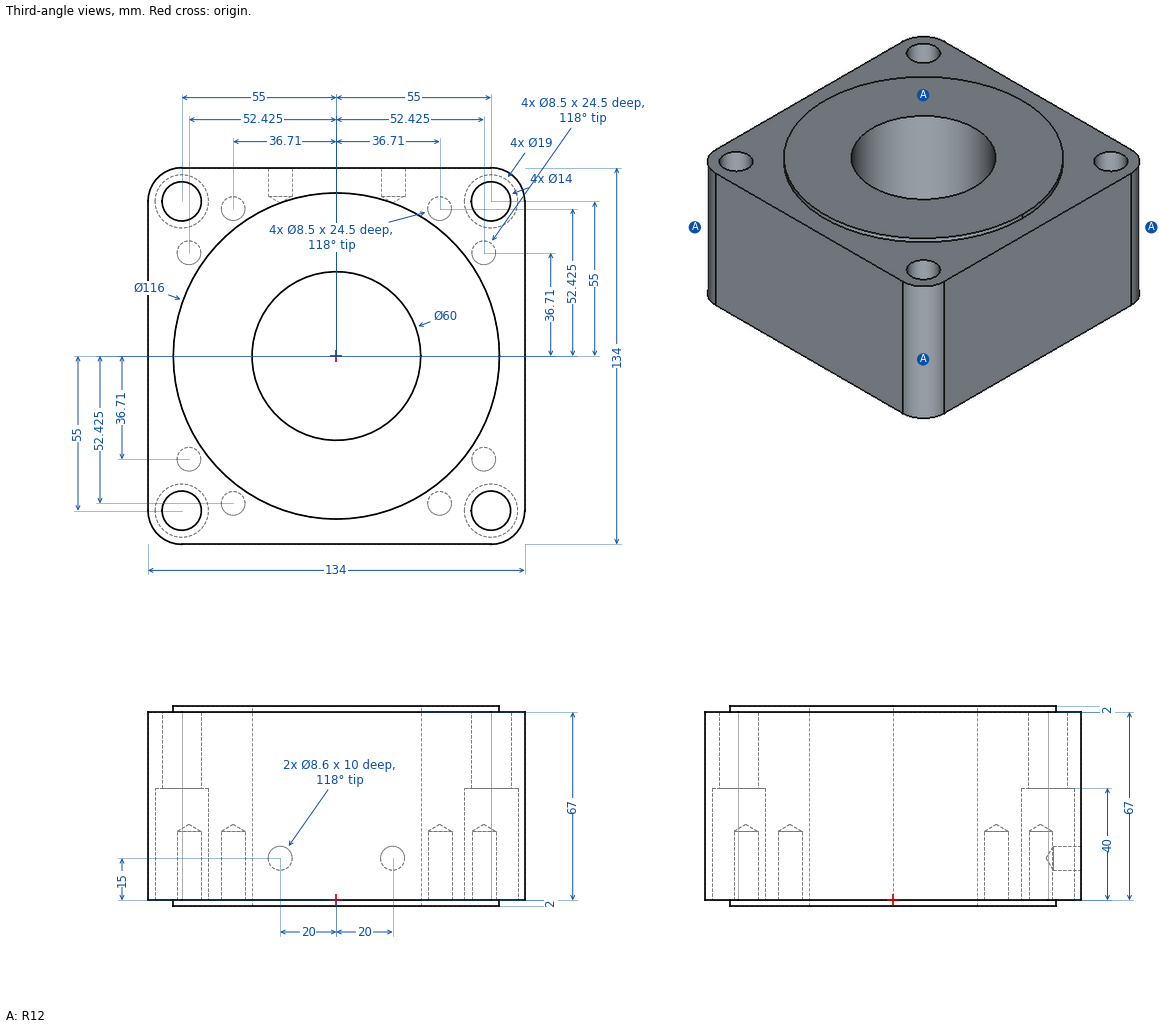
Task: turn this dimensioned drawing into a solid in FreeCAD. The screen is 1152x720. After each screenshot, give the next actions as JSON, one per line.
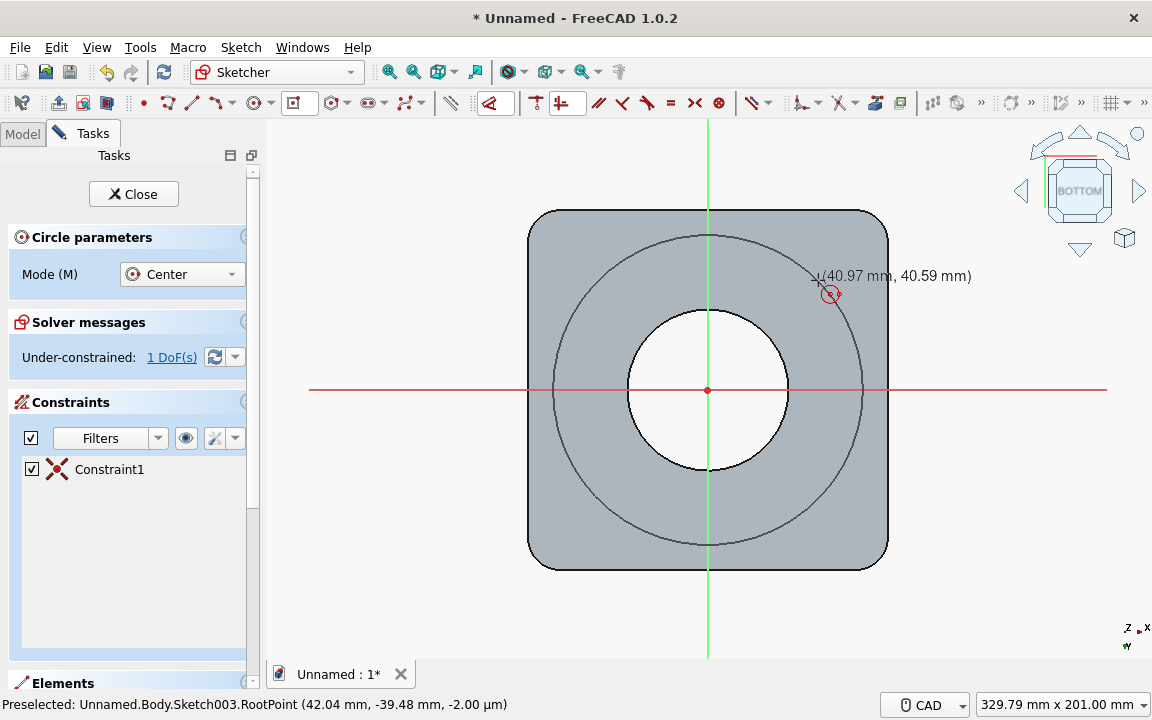
{"action": "left_click", "coordinate": [708, 390]}
{"action": "left_click", "coordinate": [765, 333]}
{"action": "key", "text": "Escape"}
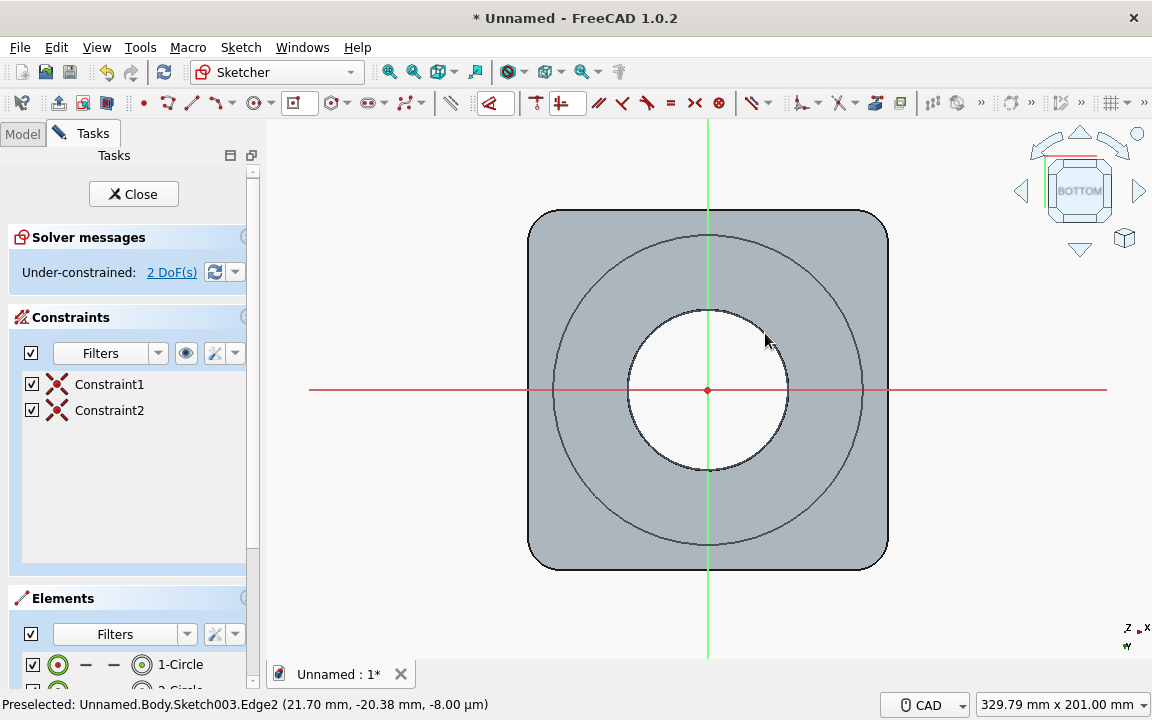
{"action": "left_click", "coordinate": [817, 280]}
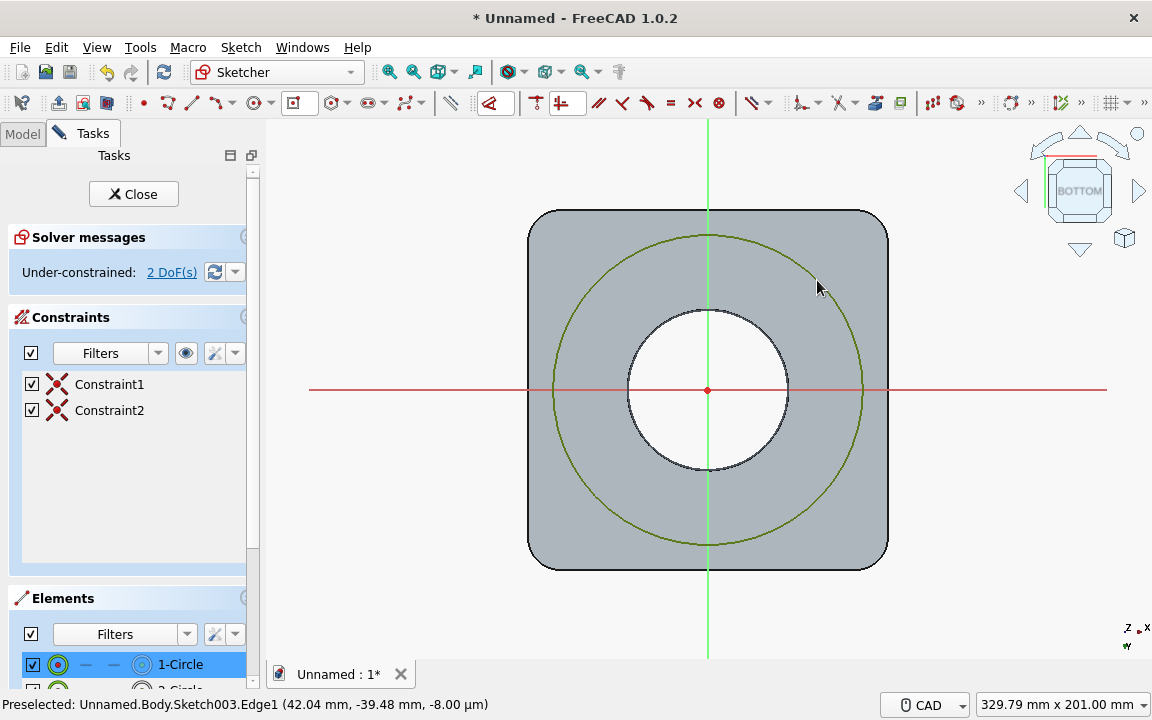
{"action": "left_click", "coordinate": [508, 104]}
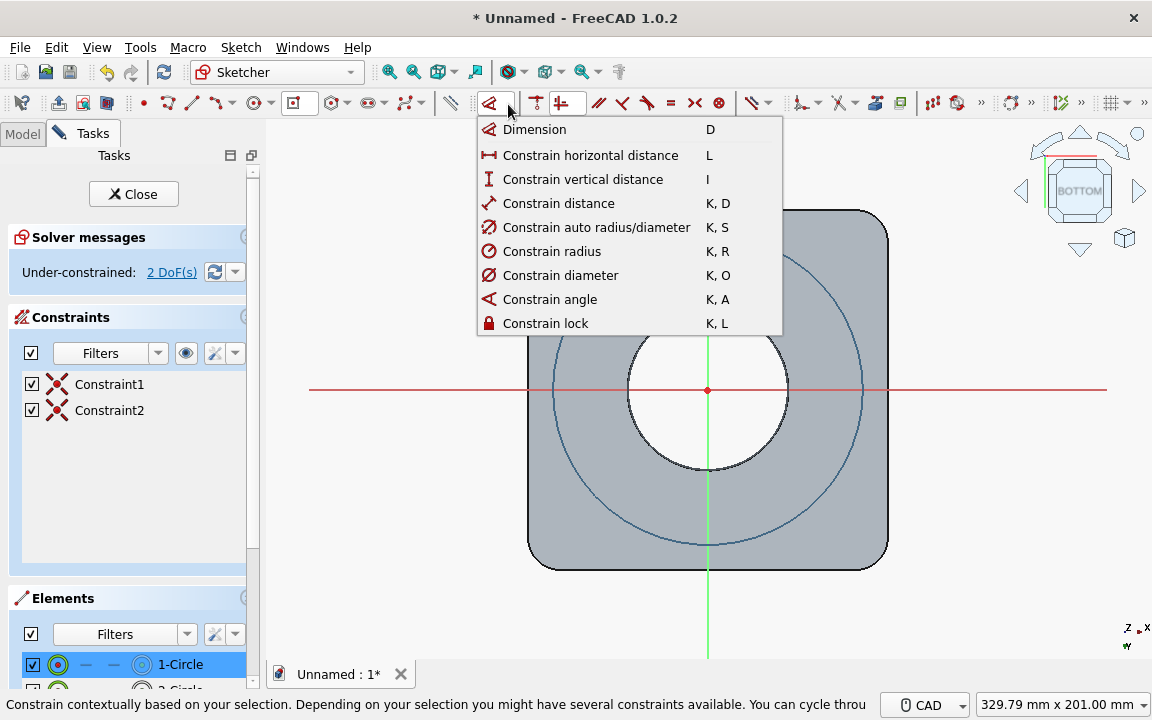
{"action": "left_click", "coordinate": [630, 275]}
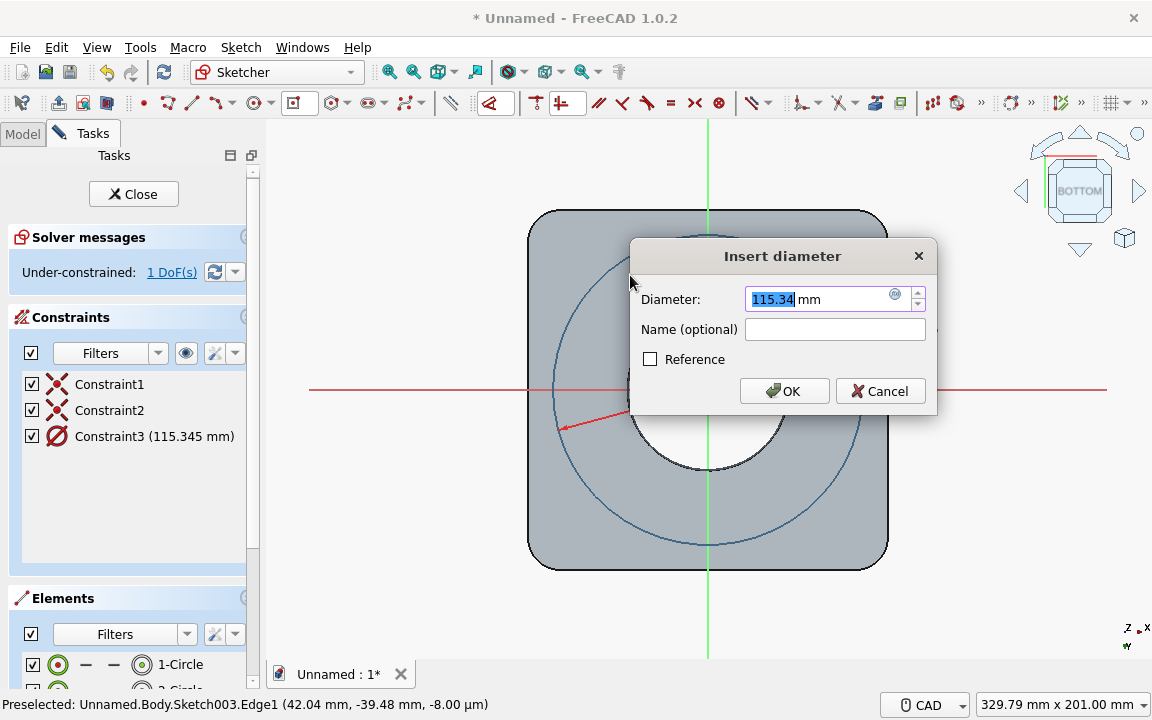
{"action": "type", "text": "116"}
{"action": "key", "text": "Return"}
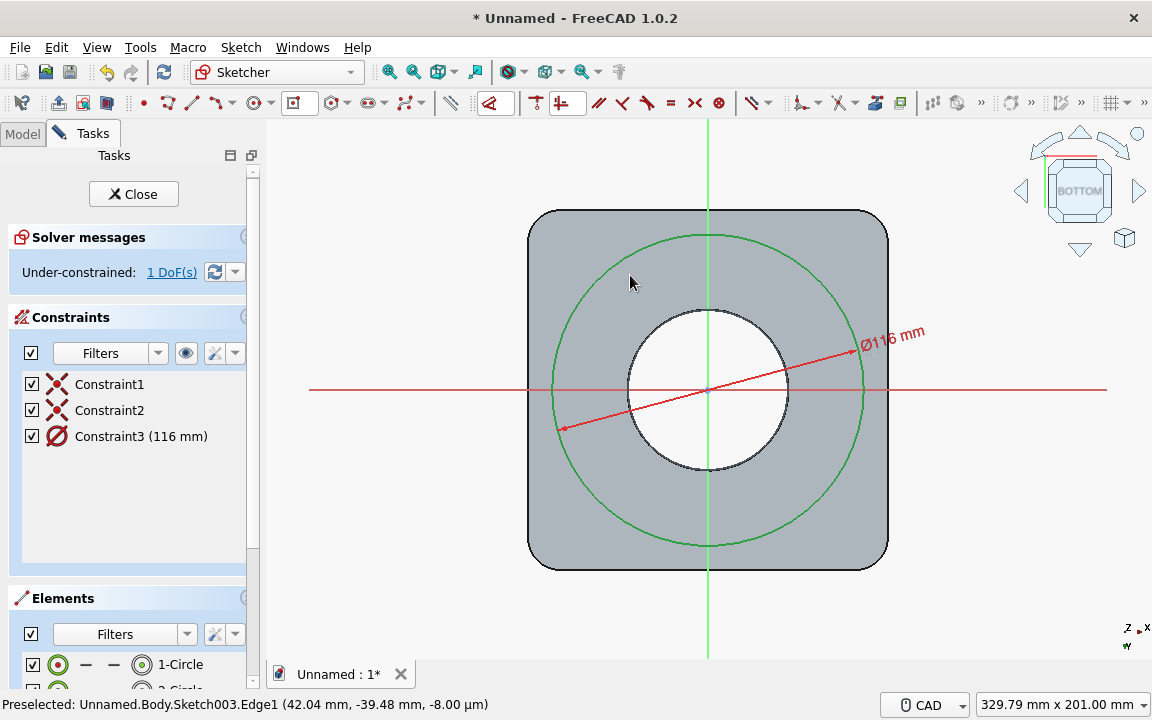
{"action": "left_click", "coordinate": [764, 333]}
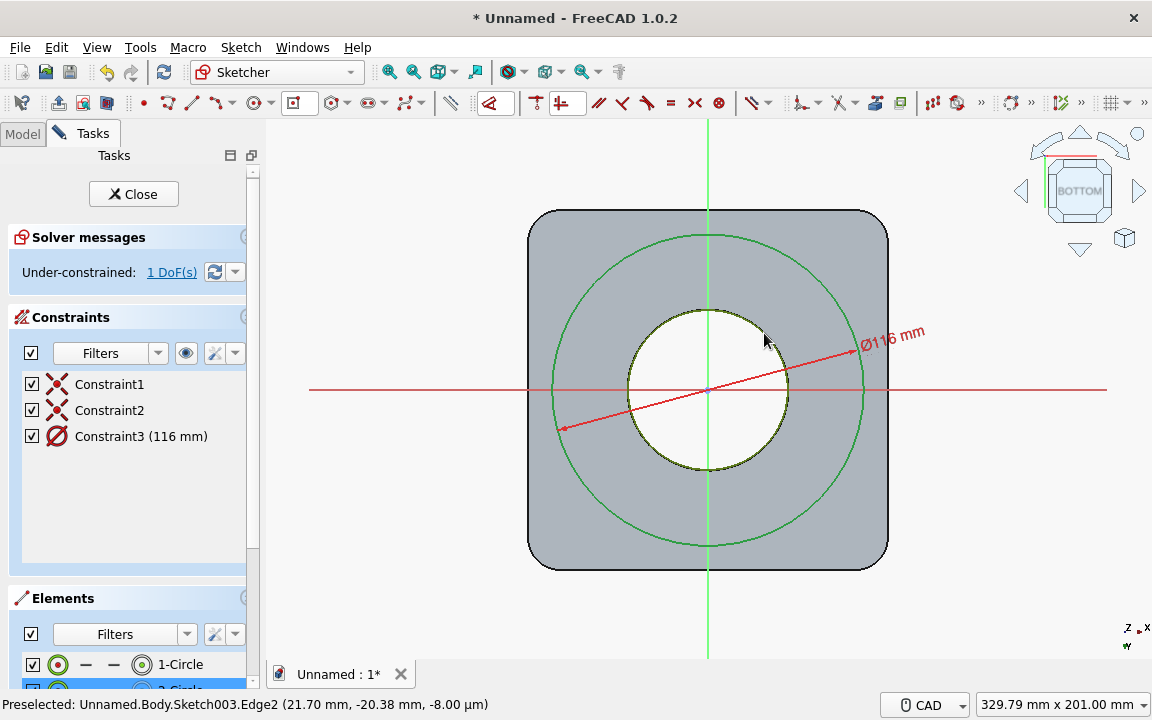
{"action": "key", "text": "k o"}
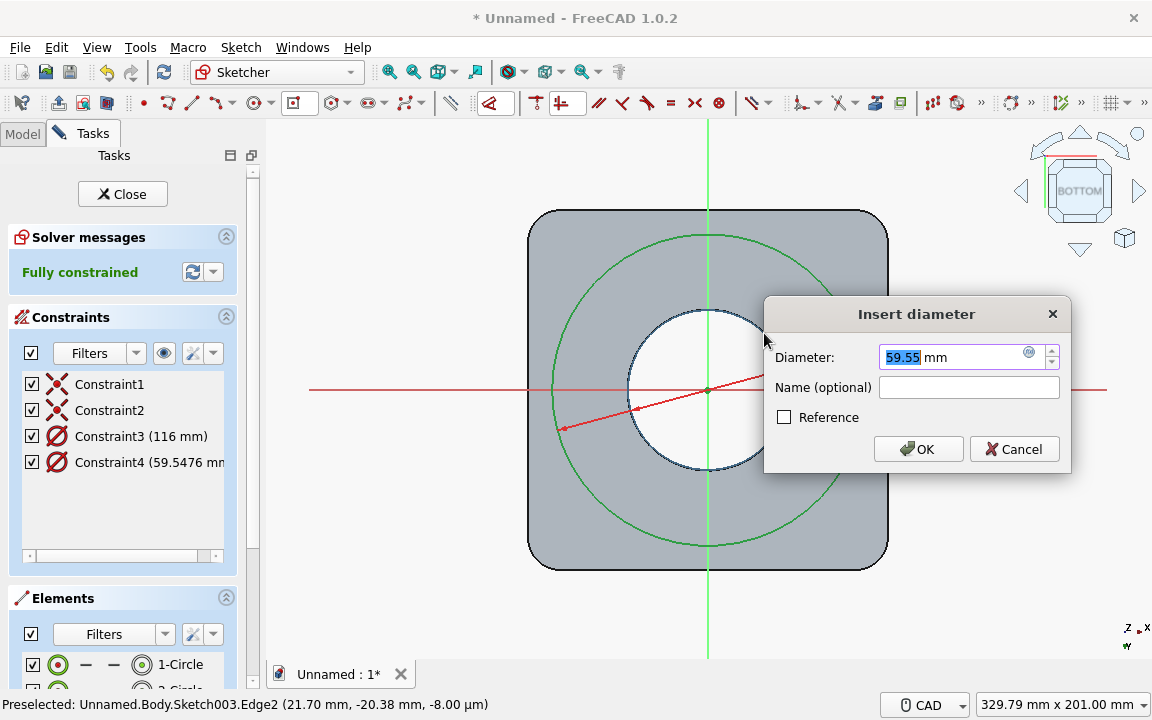
{"action": "type", "text": "60"}
{"action": "key", "text": "Return"}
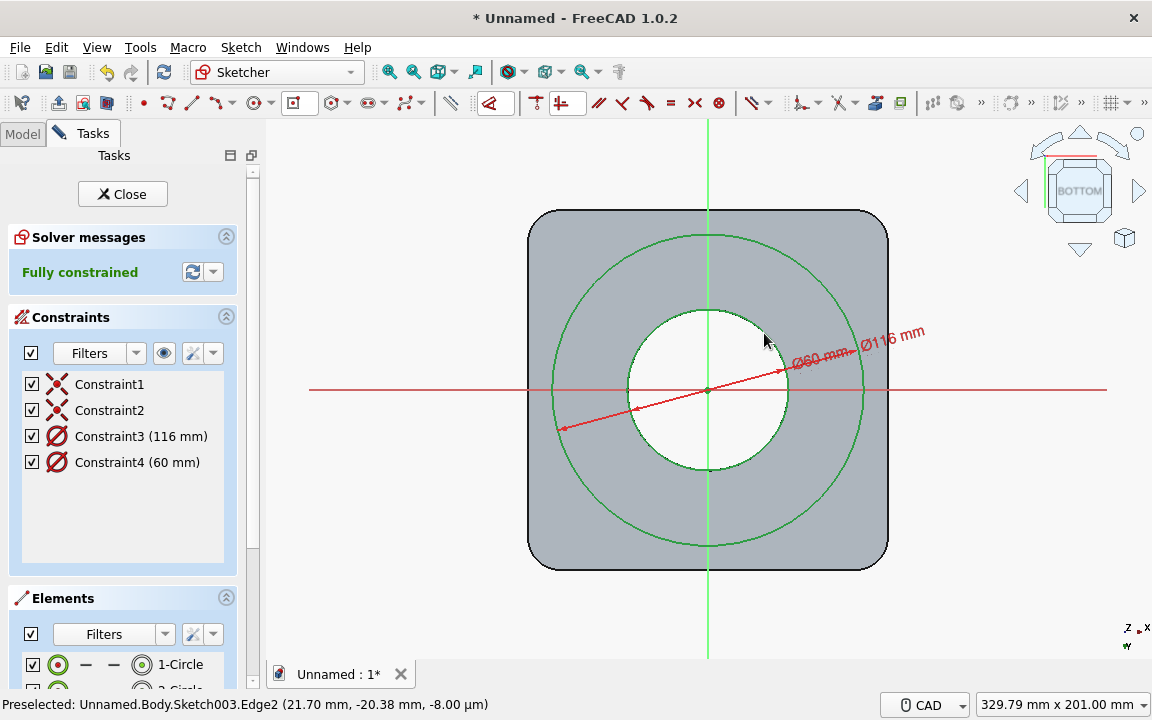
{"action": "left_click", "coordinate": [123, 194]}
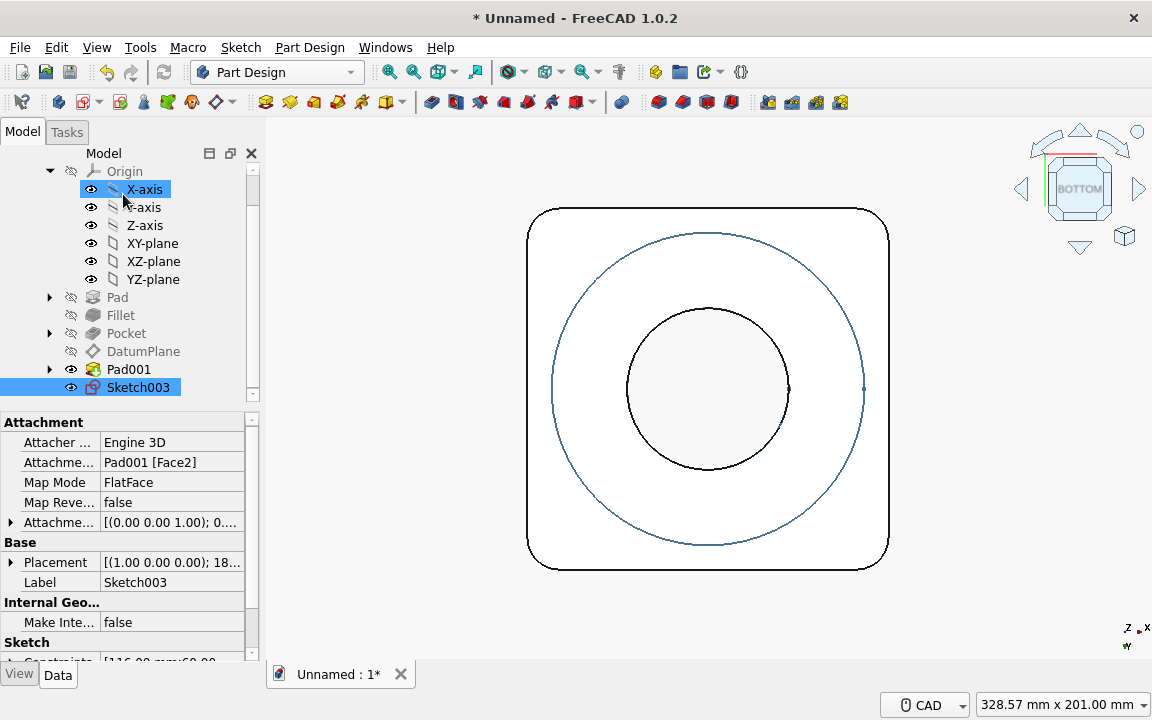
{"action": "left_click", "coordinate": [266, 102]}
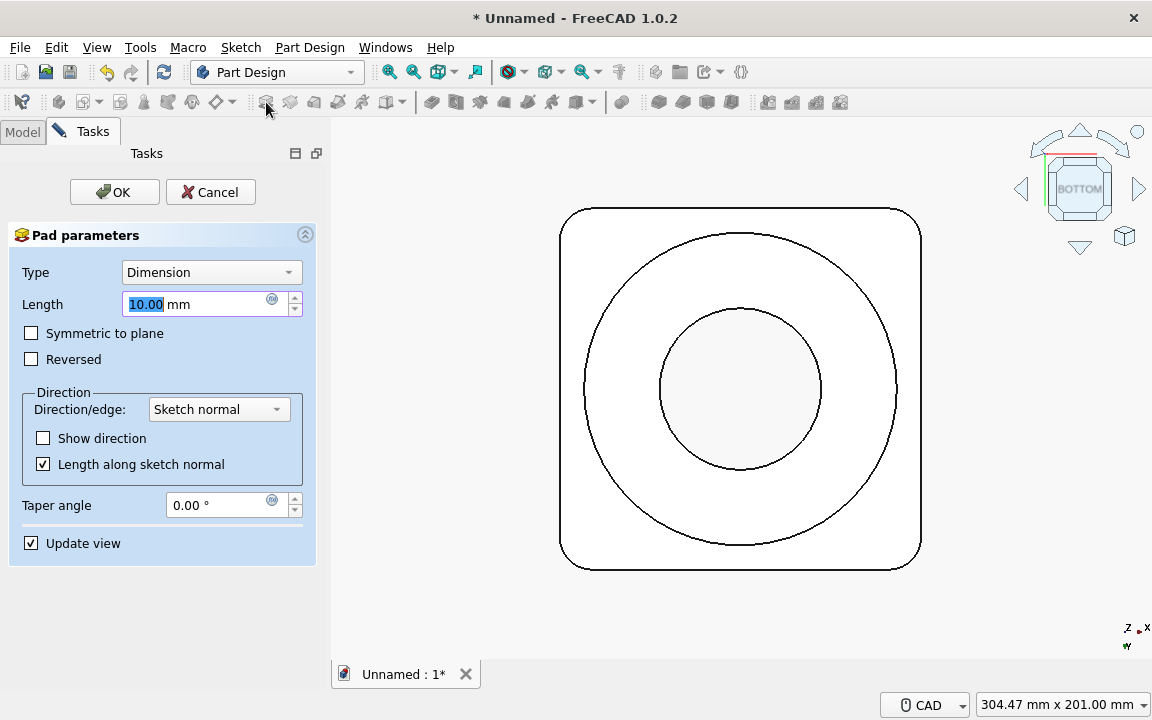
{"action": "type", "text": "2"}
{"action": "key", "text": "Tab"}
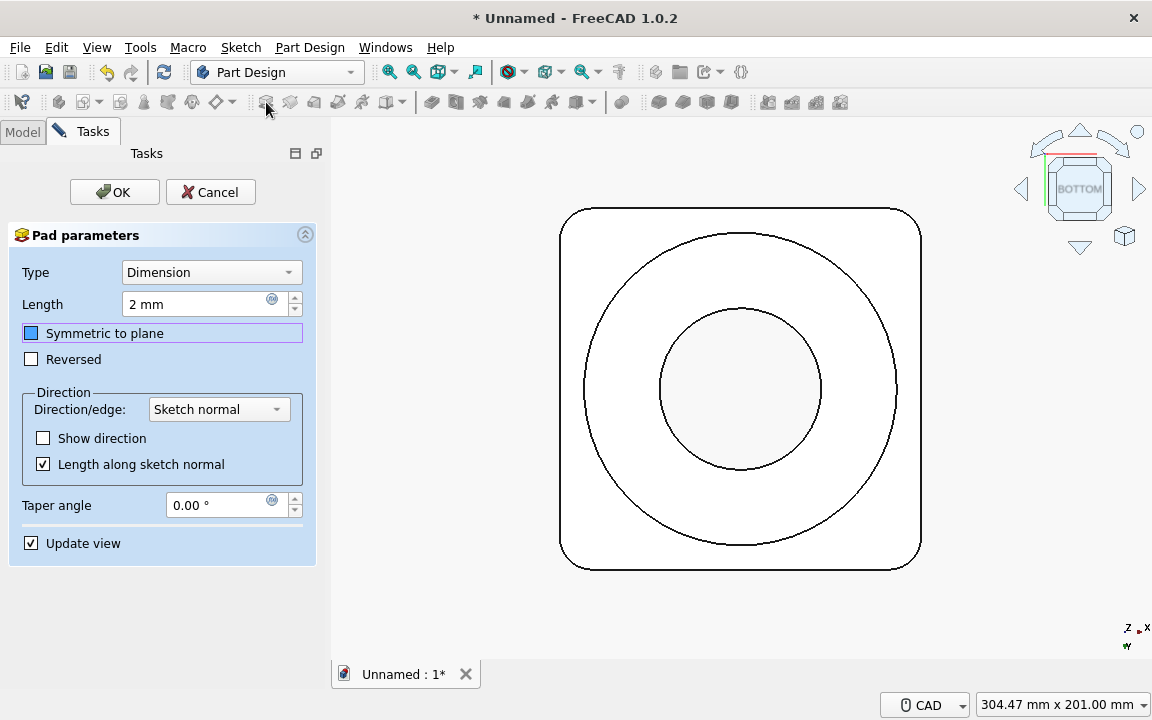
{"action": "left_click", "coordinate": [115, 192]}